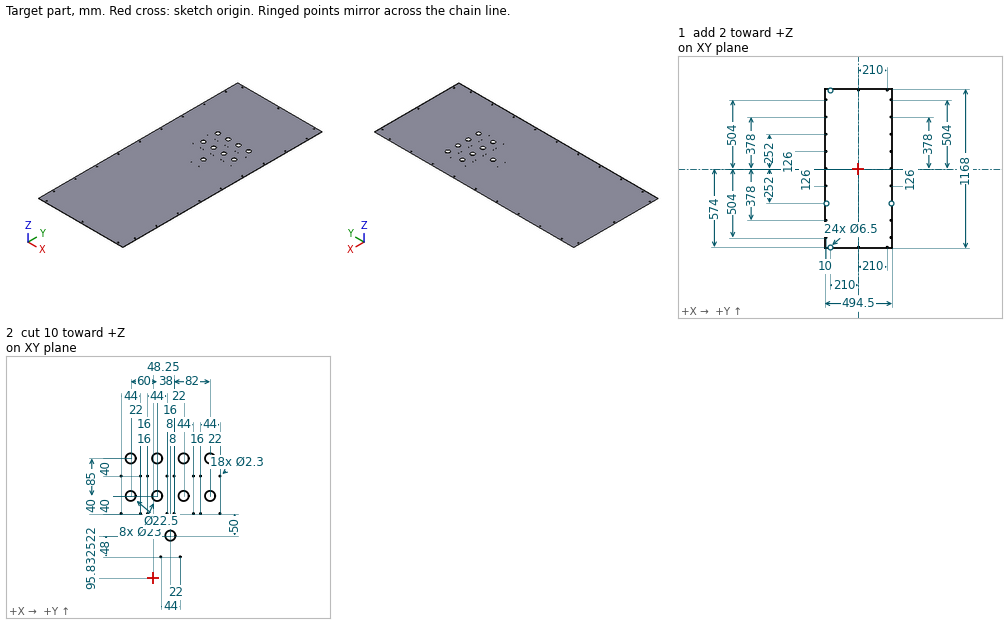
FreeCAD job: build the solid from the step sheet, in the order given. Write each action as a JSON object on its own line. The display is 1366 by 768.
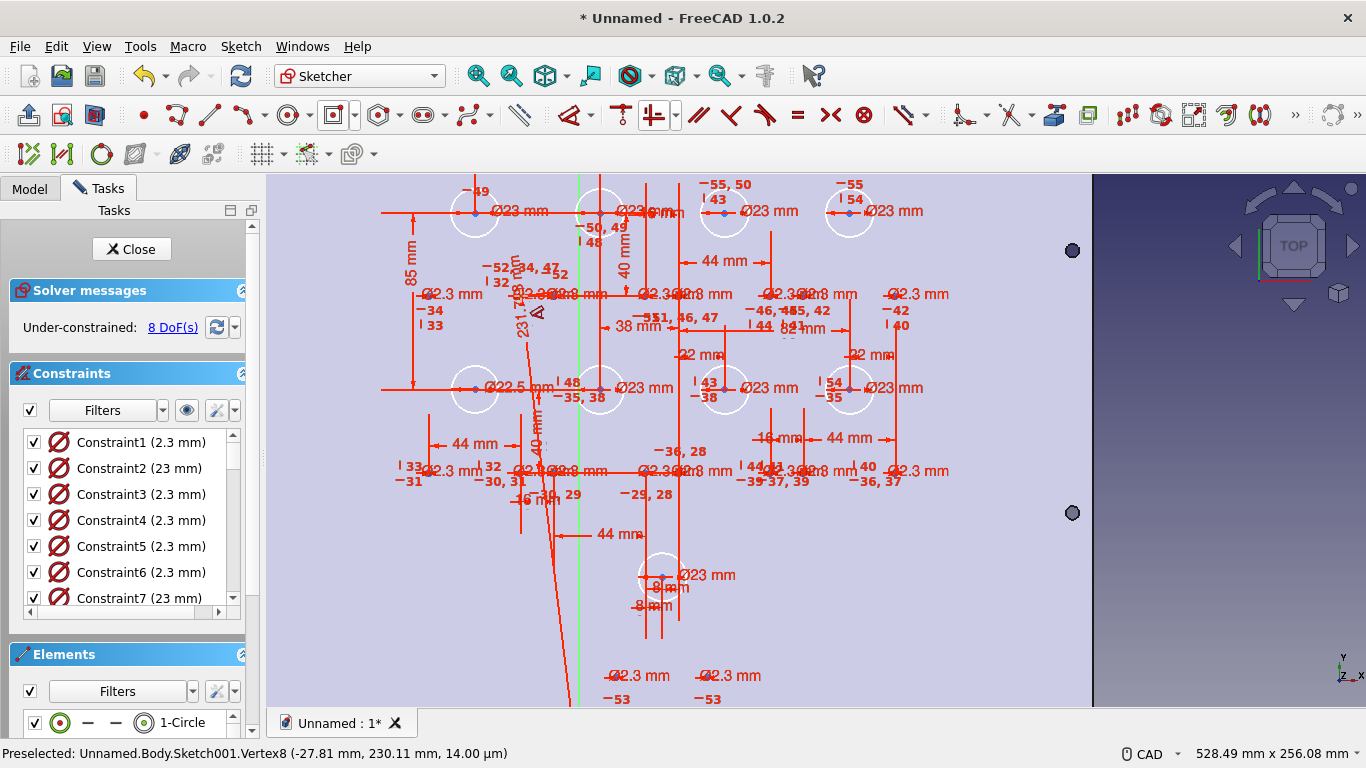
{"action": "left_click", "coordinate": [554, 296]}
{"action": "left_click", "coordinate": [538, 262]}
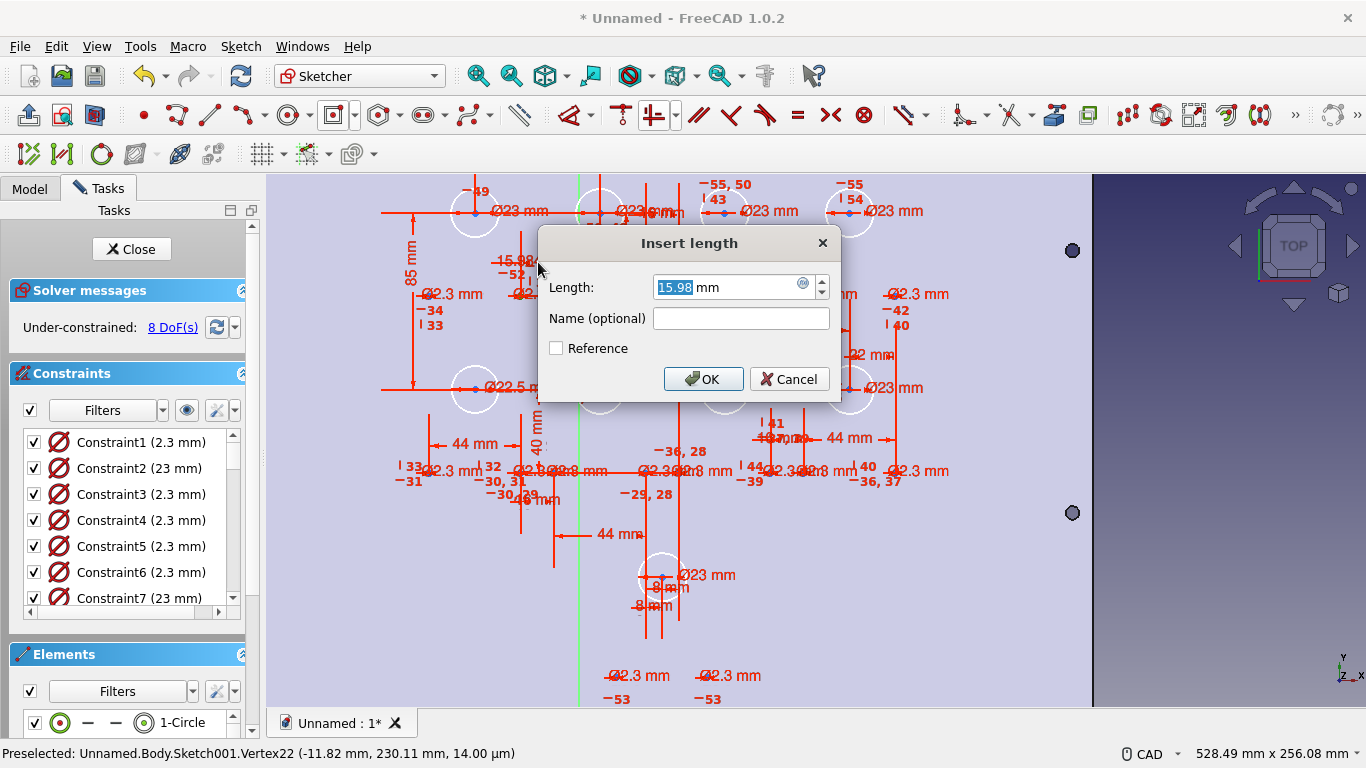
{"action": "type", "text": "16"}
{"action": "key", "text": "Return"}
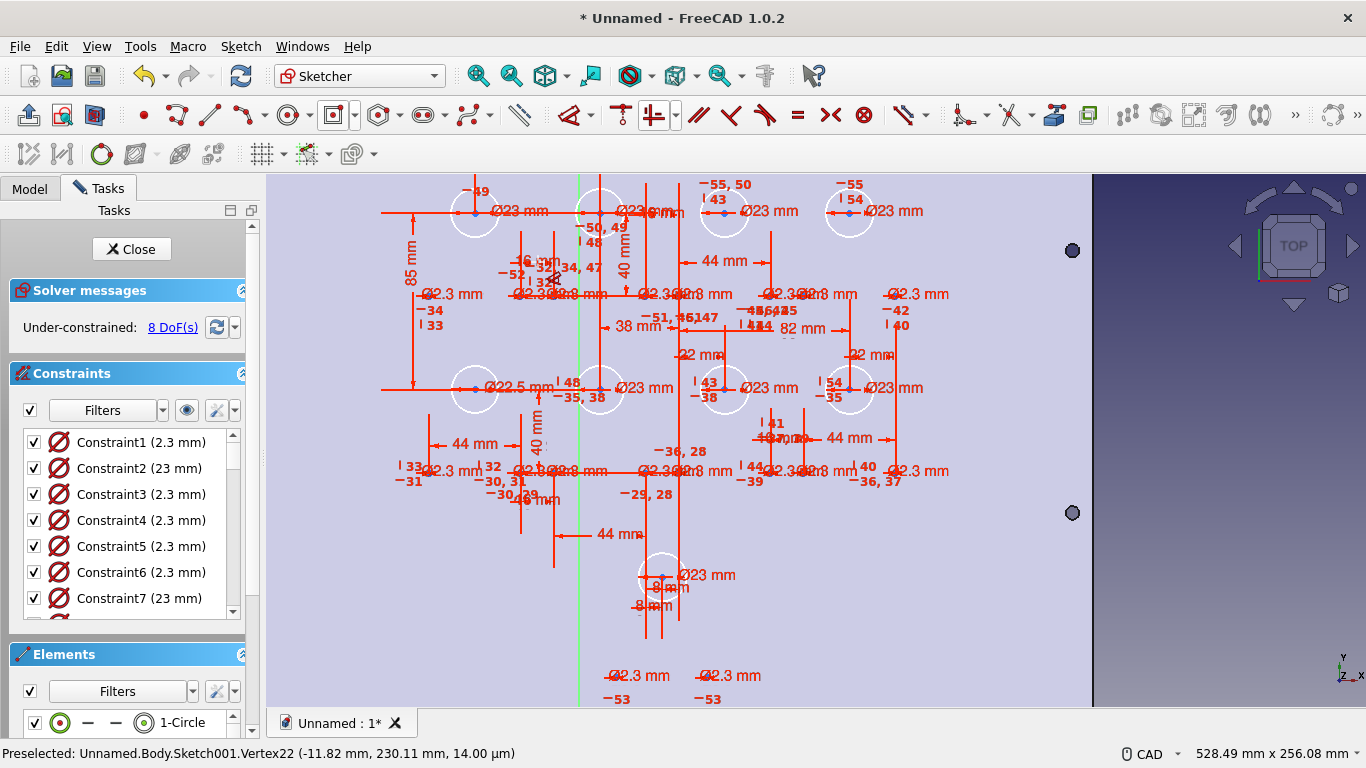
{"action": "left_click", "coordinate": [679, 473]}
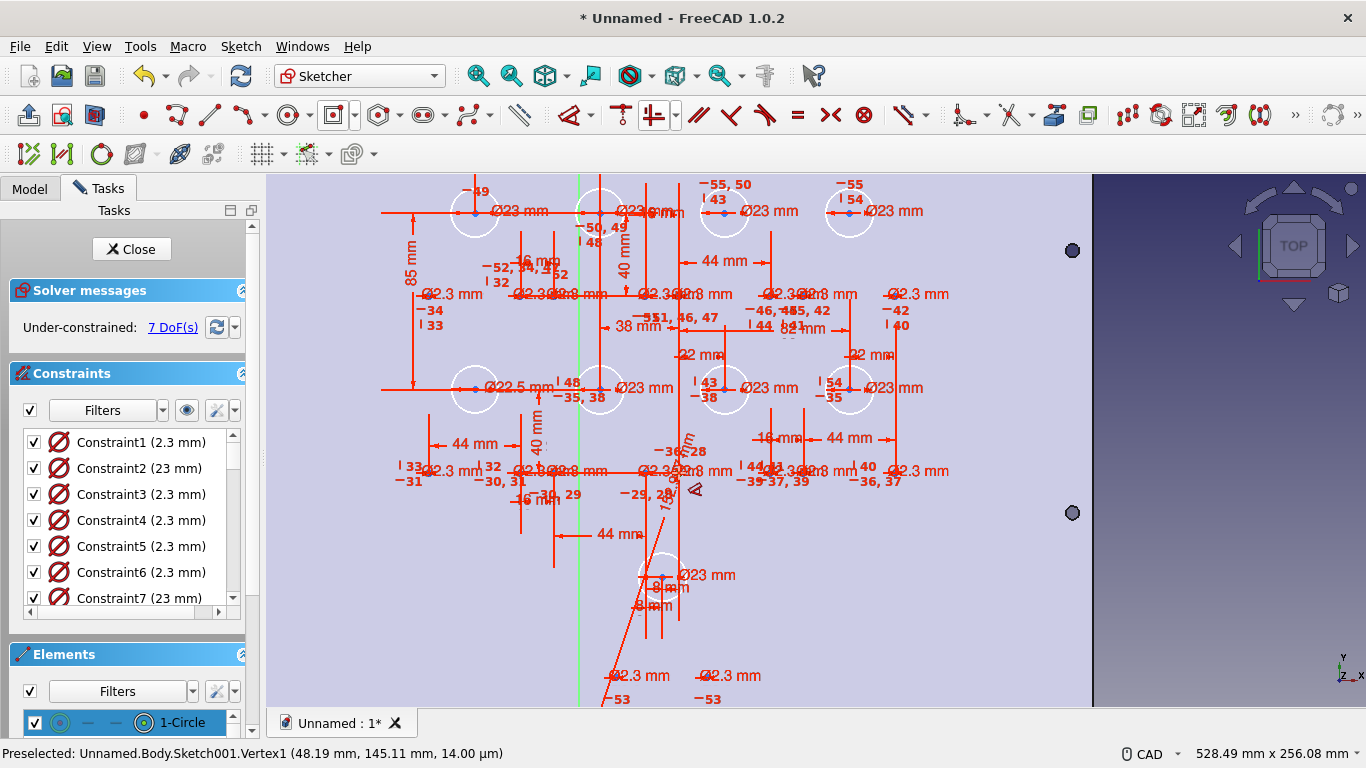
{"action": "left_click", "coordinate": [662, 577]}
{"action": "left_click", "coordinate": [713, 525]}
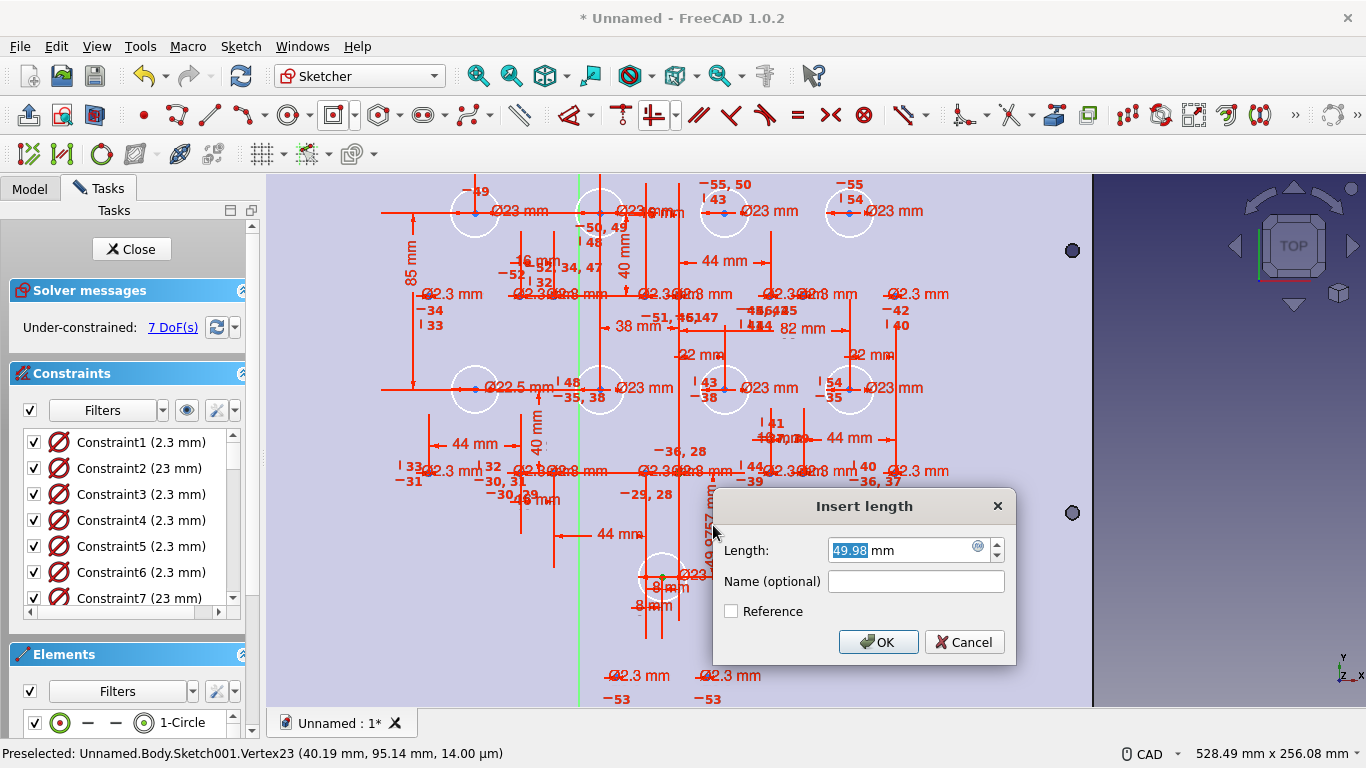
{"action": "type", "text": "50"}
{"action": "key", "text": "Return"}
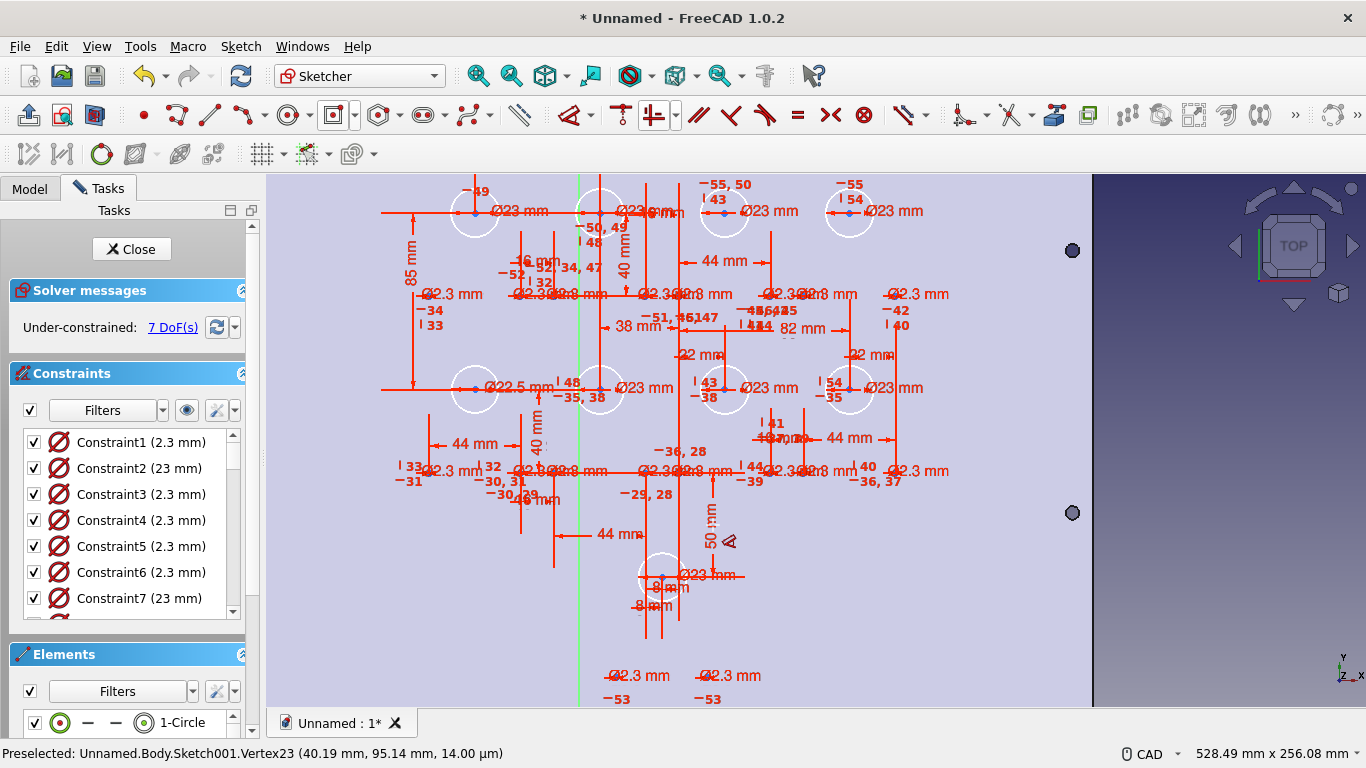
{"action": "left_click", "coordinate": [662, 577]}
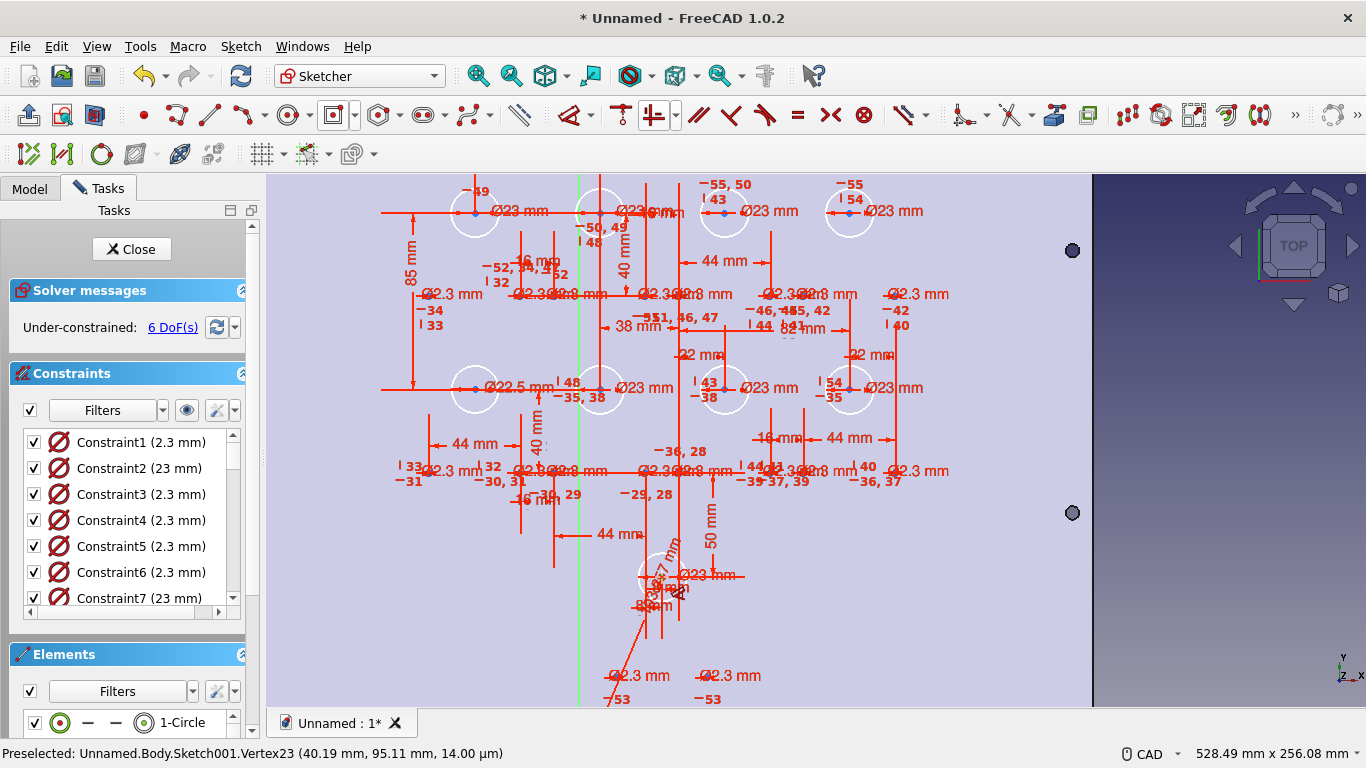
{"action": "left_click", "coordinate": [708, 678]}
{"action": "left_click", "coordinate": [685, 495]}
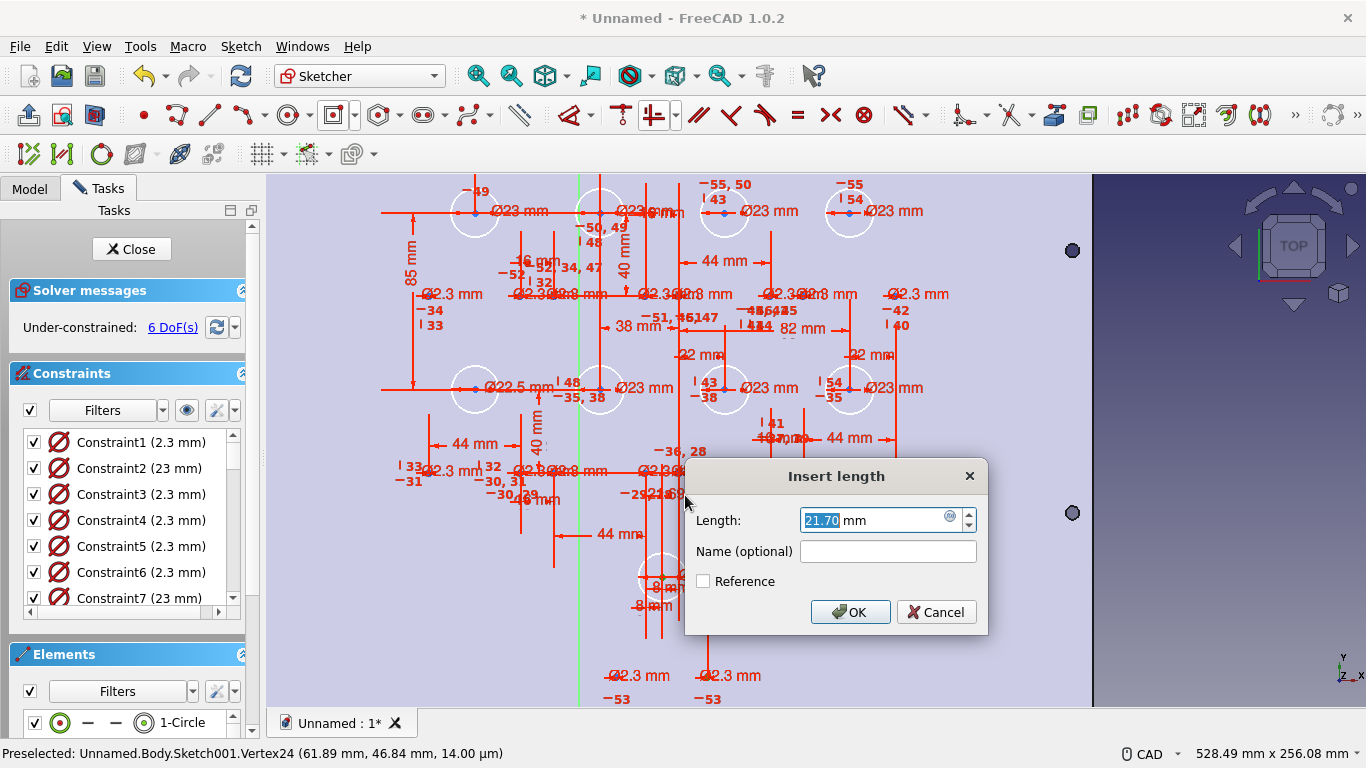
{"action": "type", "text": "22"}
{"action": "key", "text": "Return"}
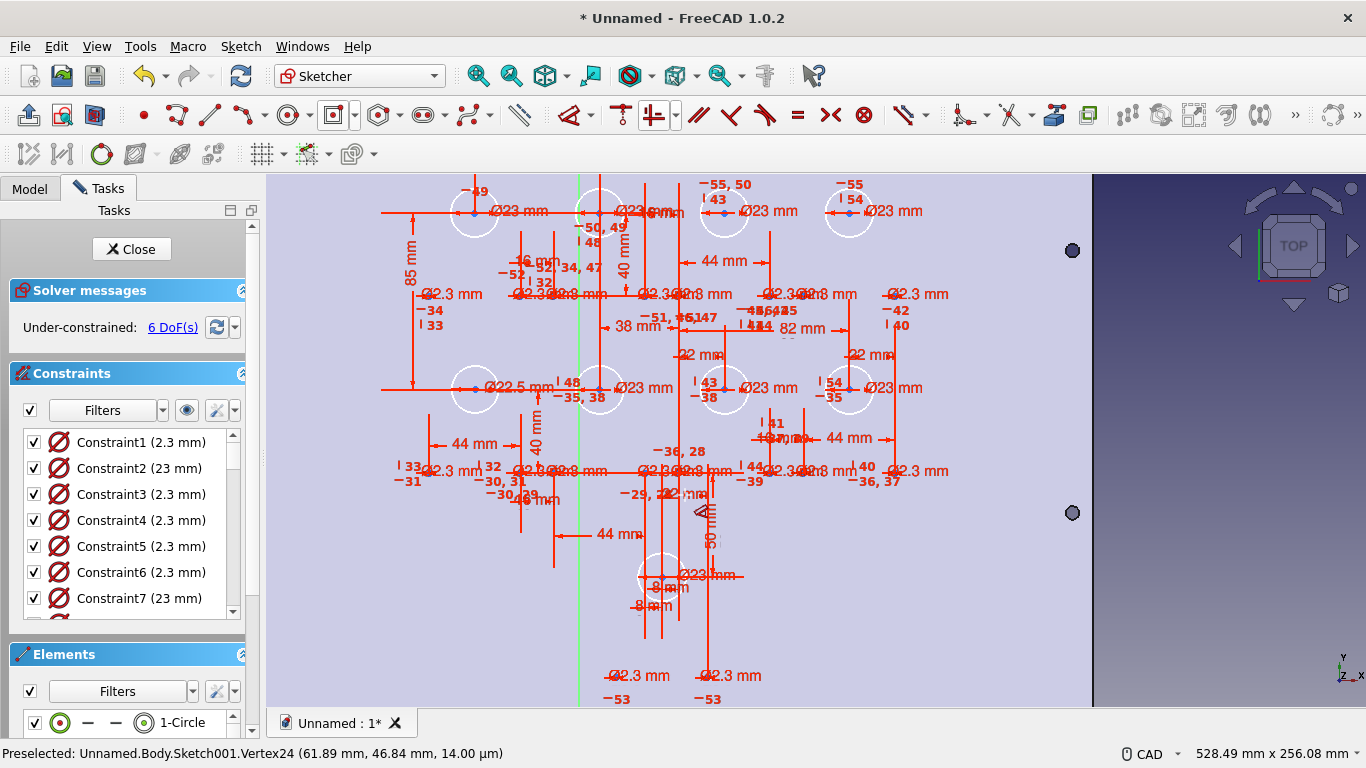
{"action": "left_click", "coordinate": [662, 577]}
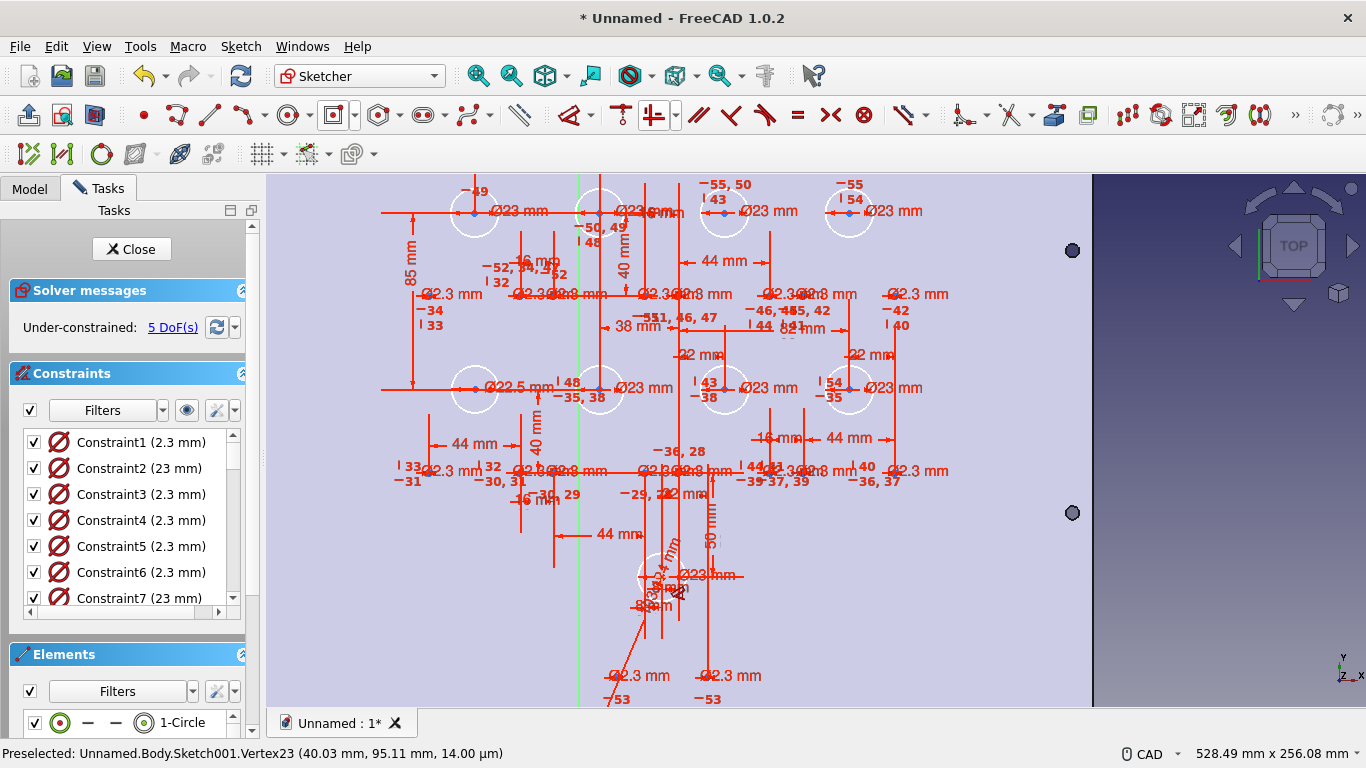
{"action": "left_click", "coordinate": [708, 678]}
{"action": "left_click", "coordinate": [742, 627]}